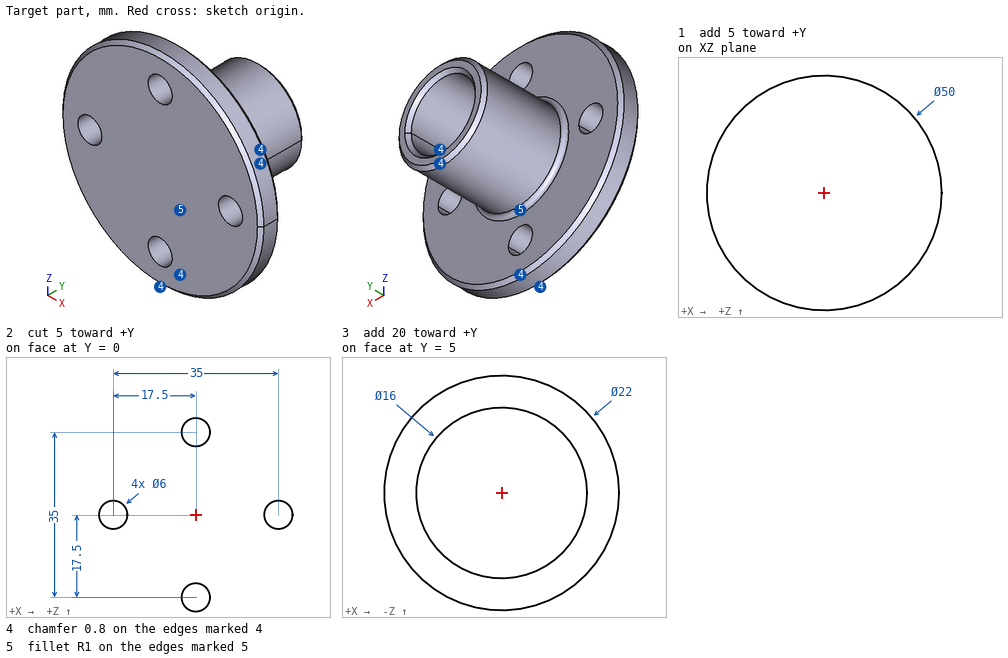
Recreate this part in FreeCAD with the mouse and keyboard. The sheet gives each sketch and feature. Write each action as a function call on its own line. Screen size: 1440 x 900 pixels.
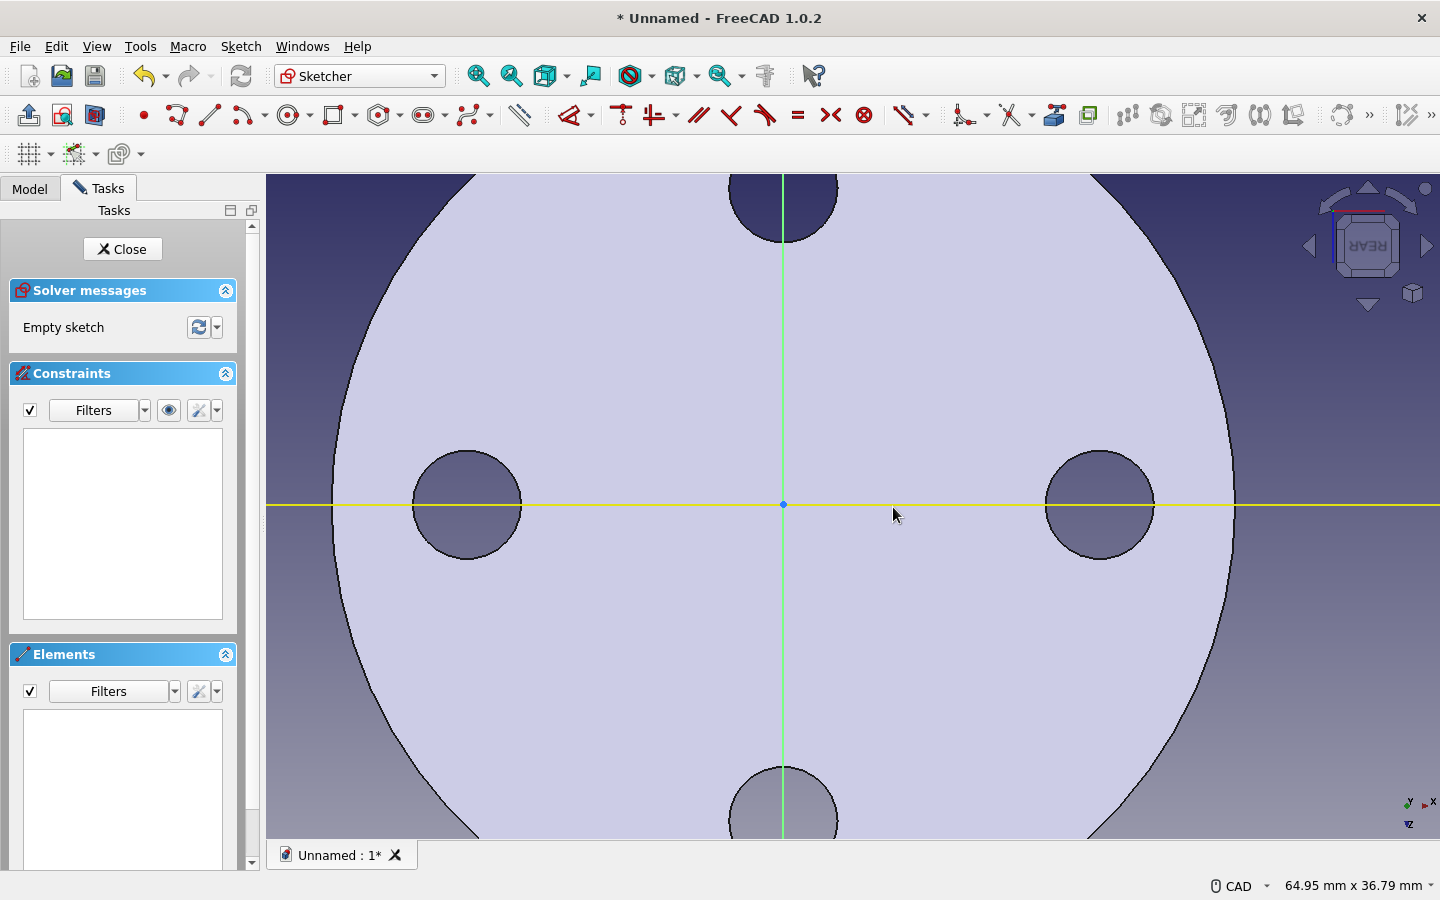
click(288, 116)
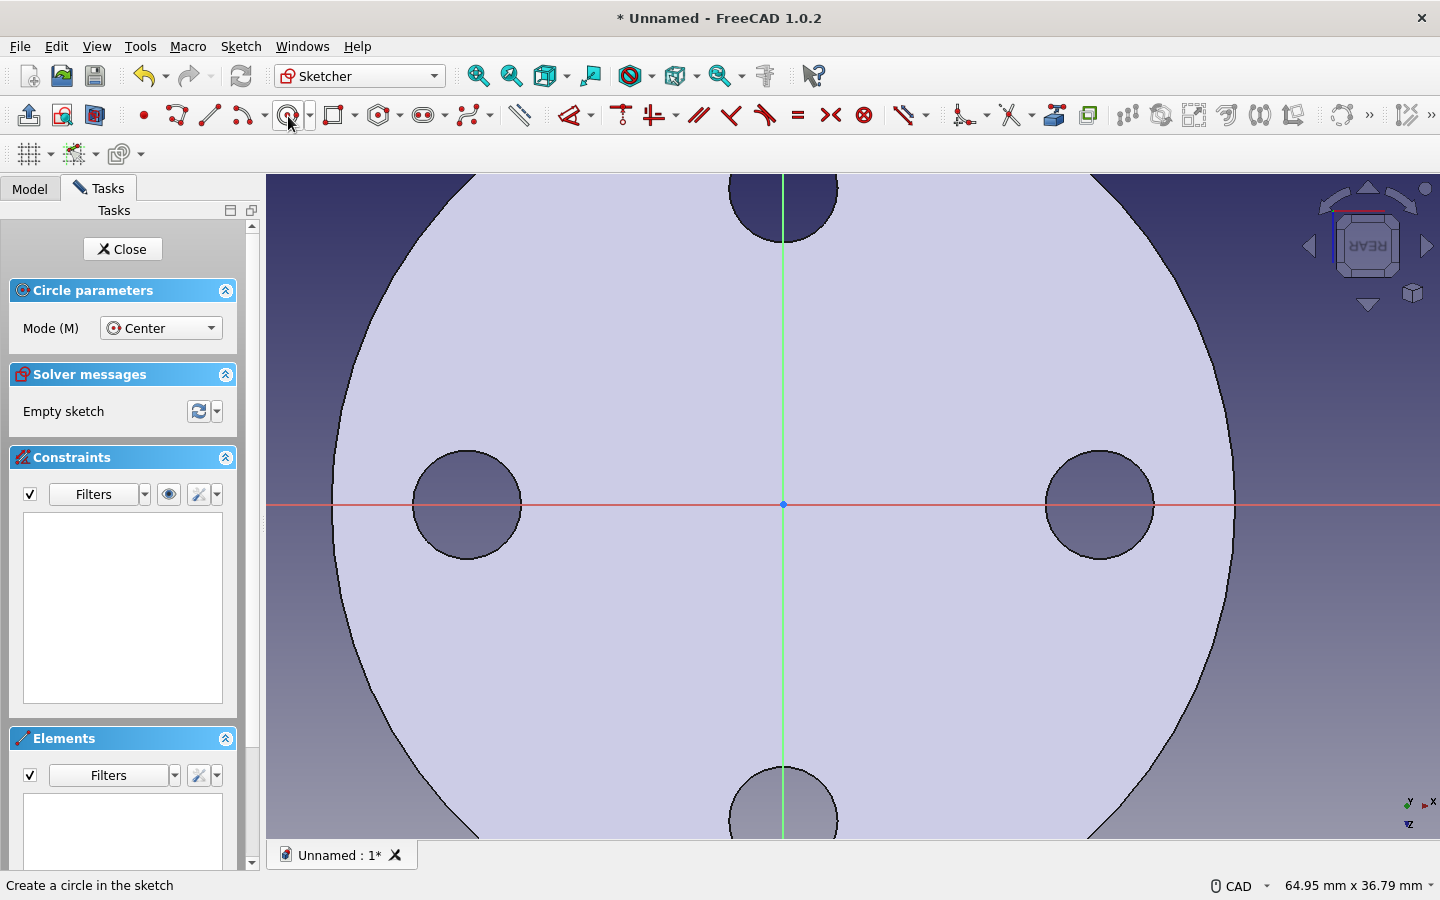
click(783, 505)
click(924, 364)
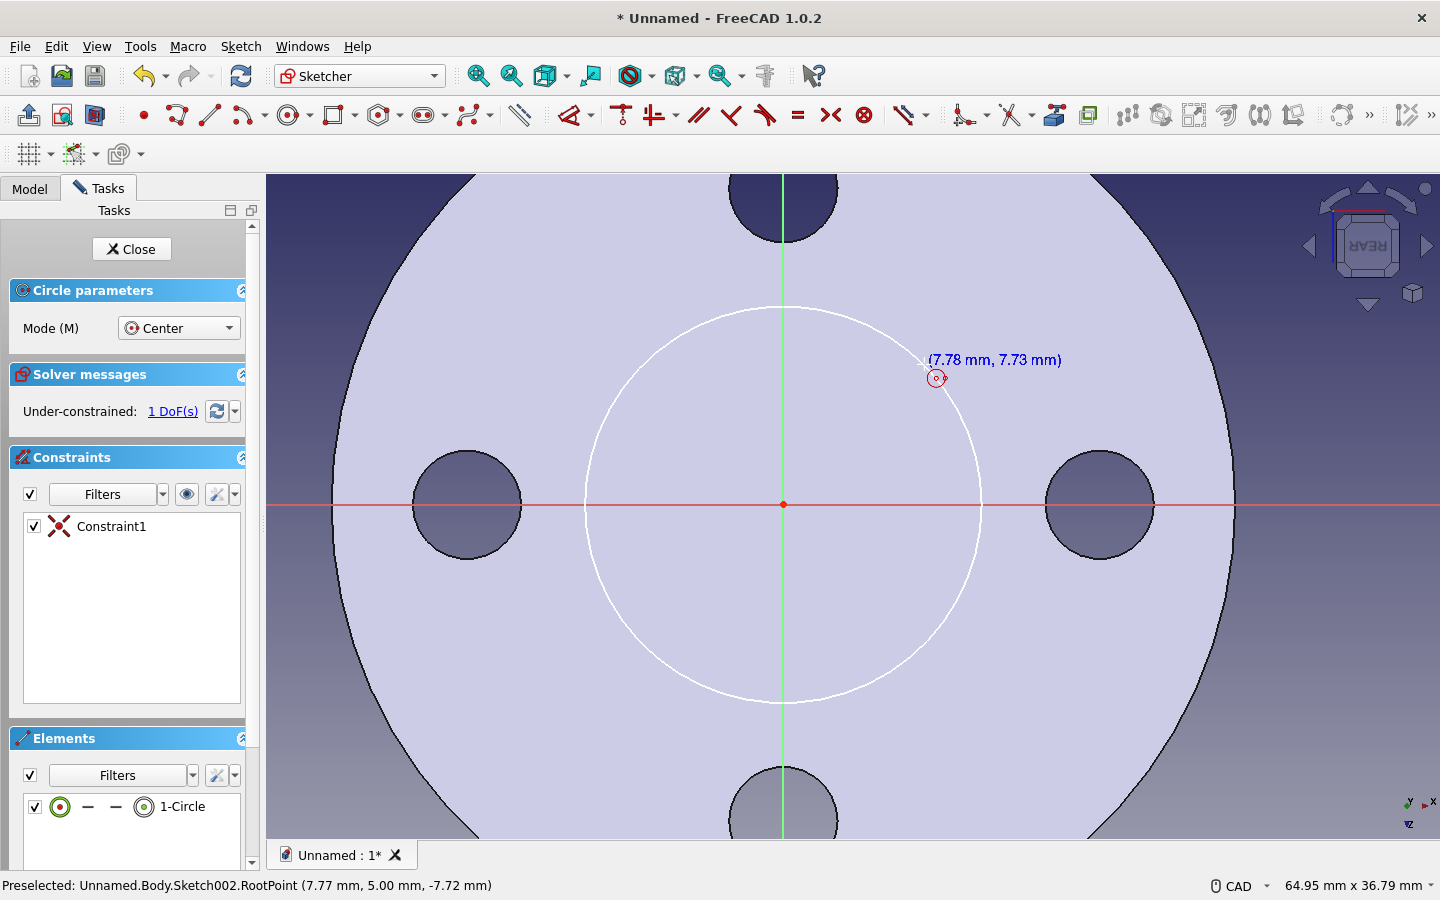
click(783, 505)
click(886, 403)
key(Escape)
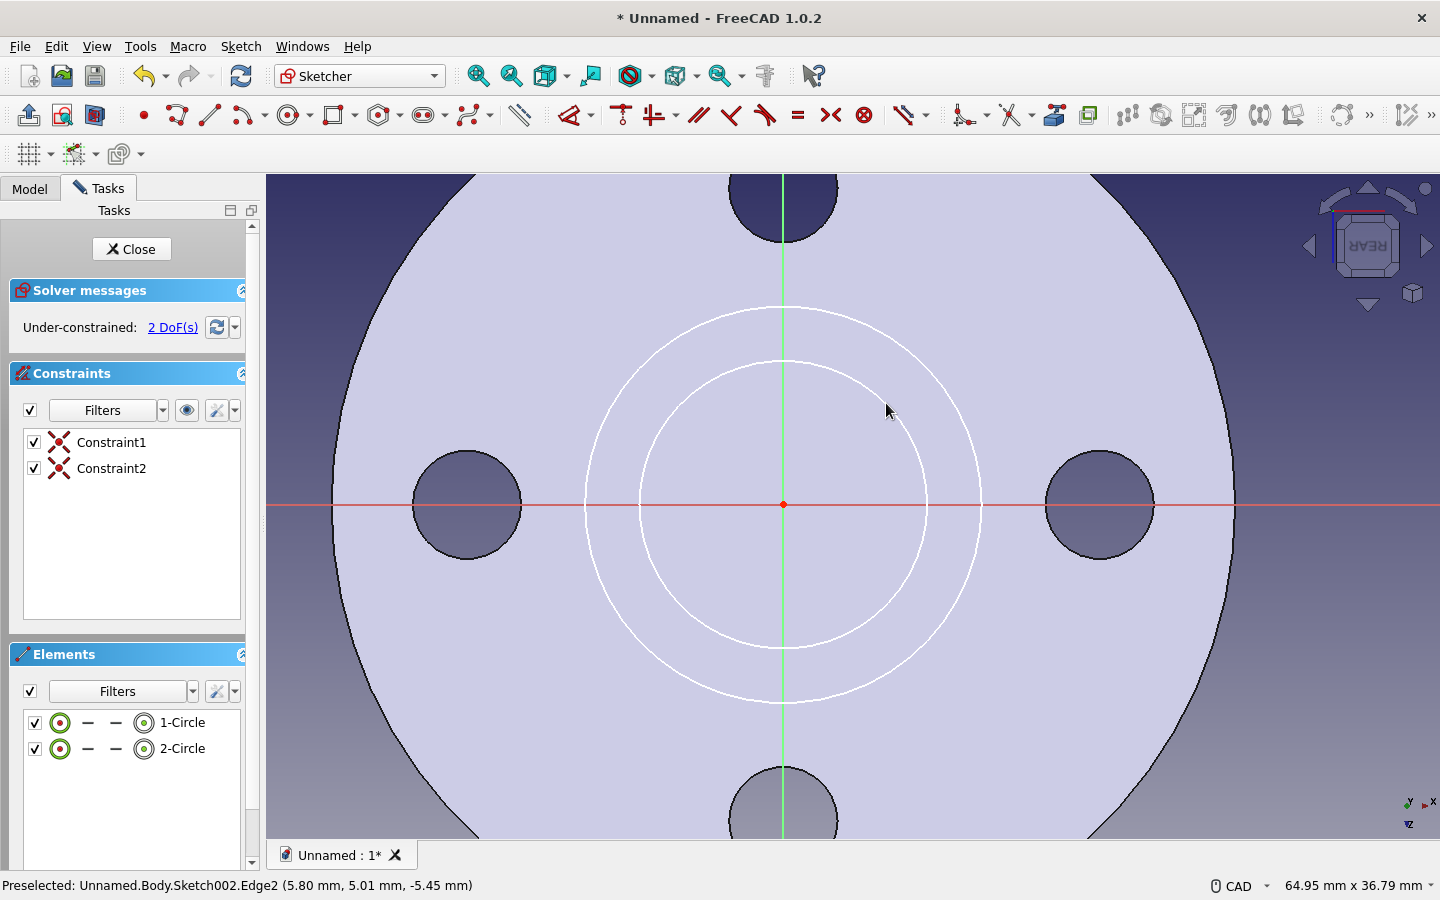
click(568, 116)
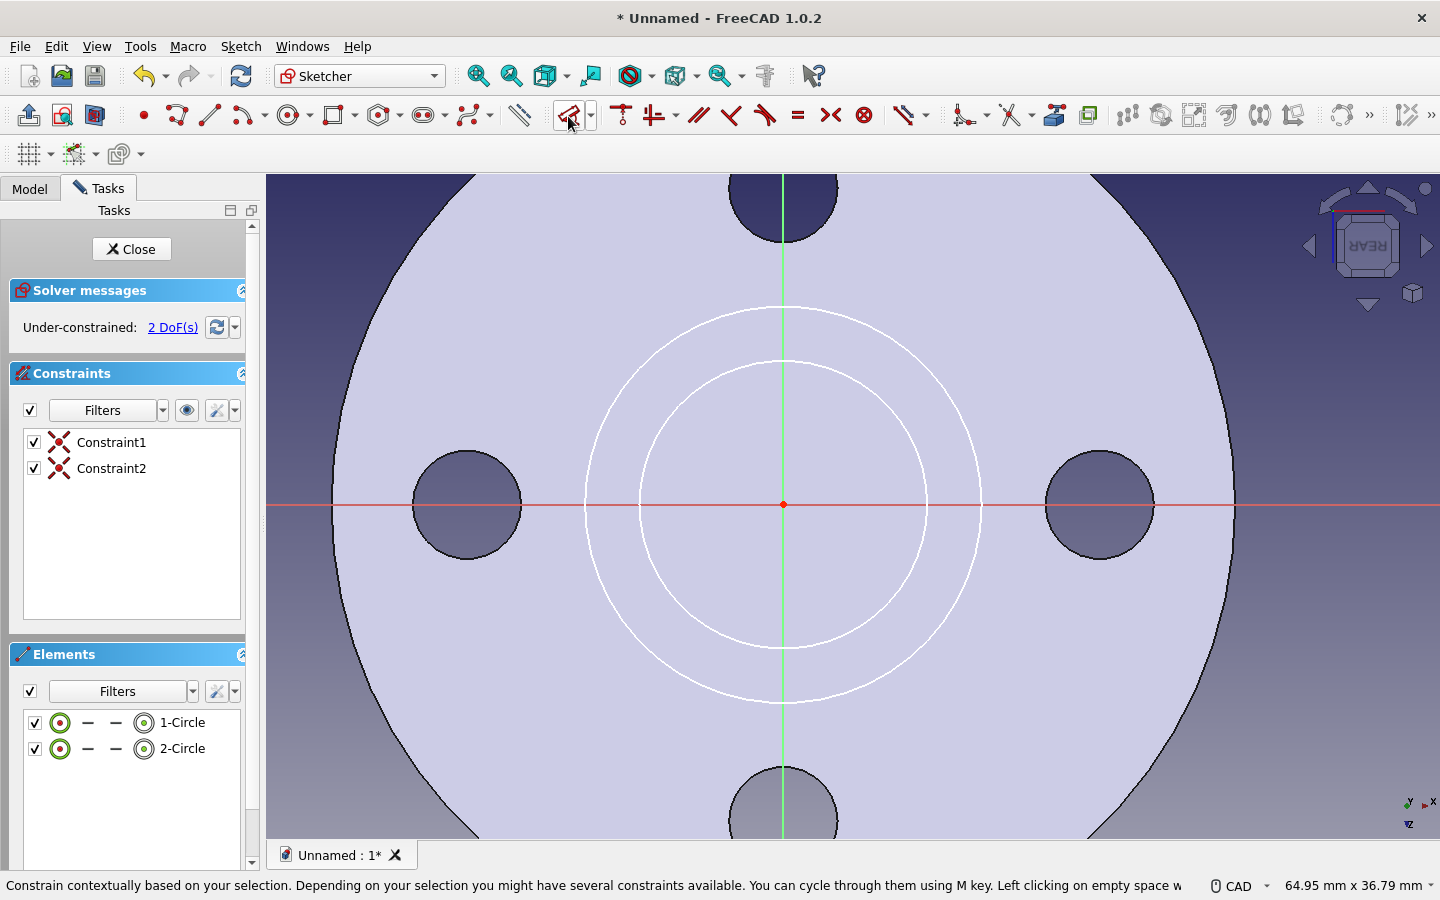
click(923, 364)
click(946, 341)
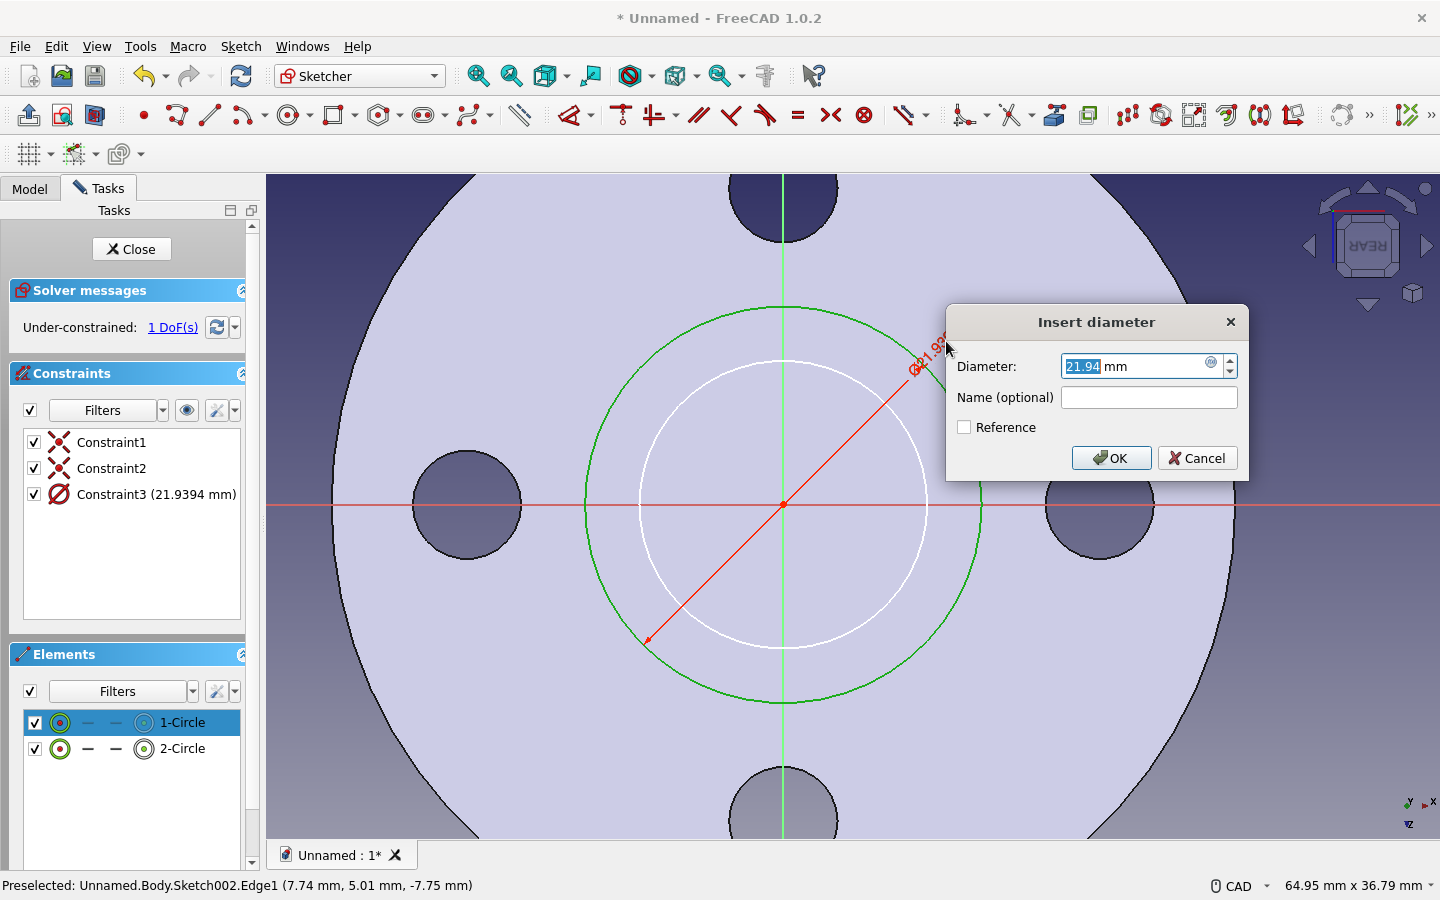
text(22)
key(Return)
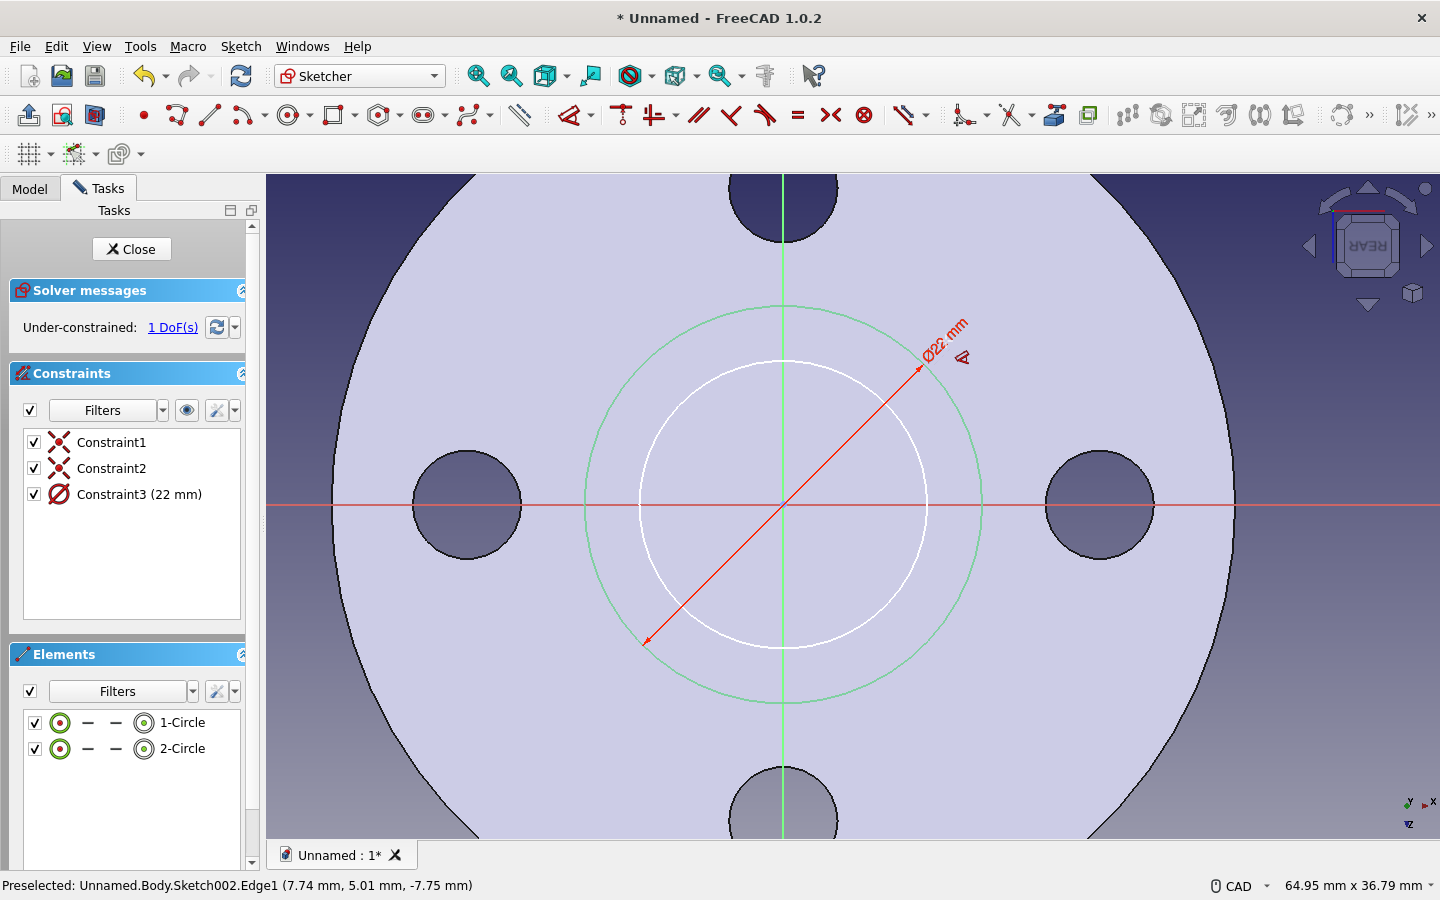
click(885, 403)
click(908, 380)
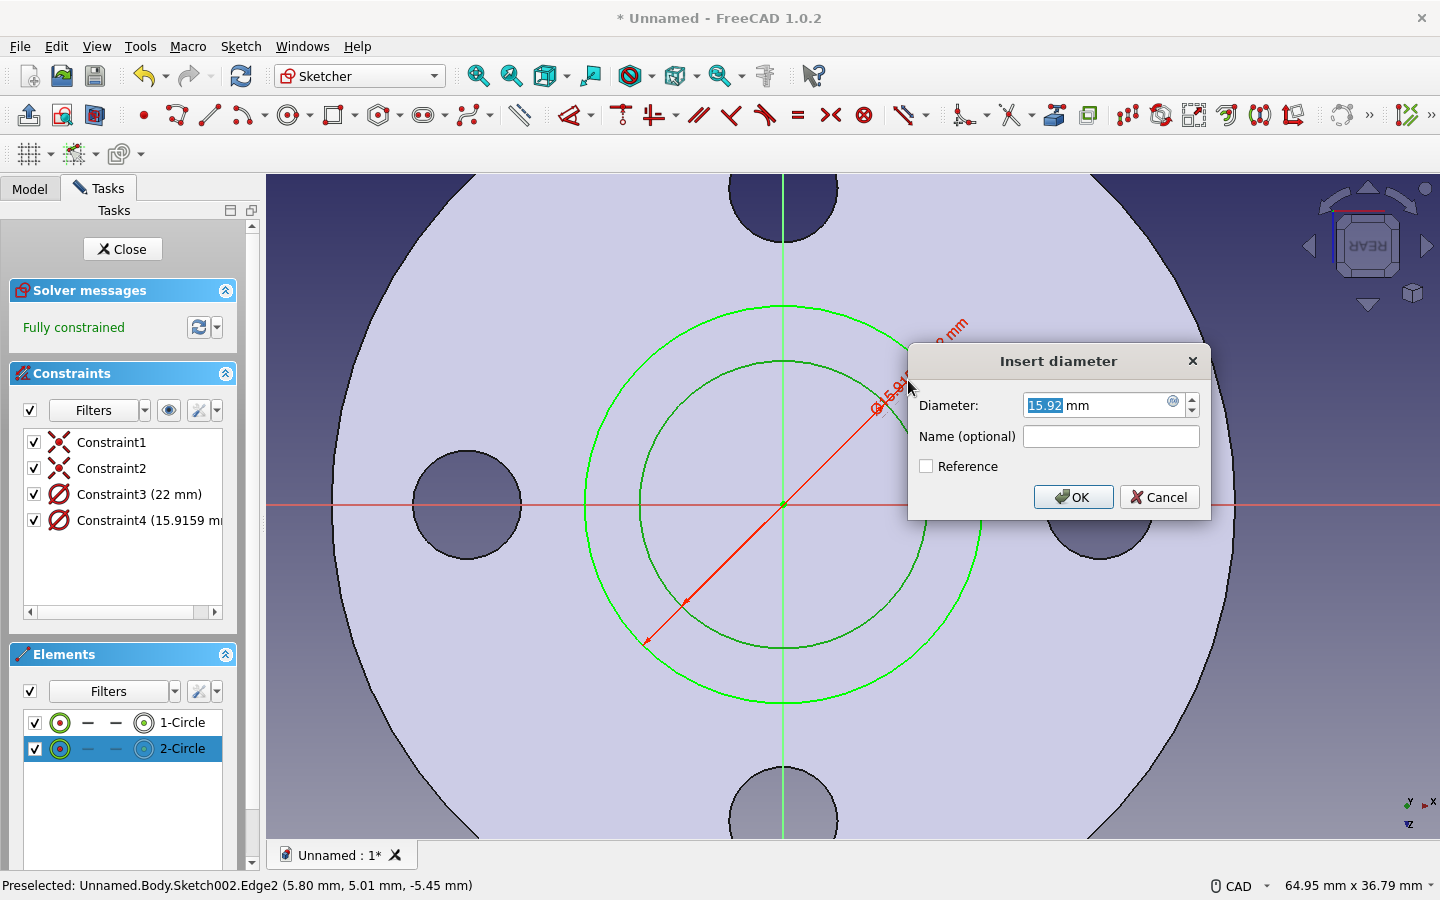
text(16)
key(Return)
key(Escape)